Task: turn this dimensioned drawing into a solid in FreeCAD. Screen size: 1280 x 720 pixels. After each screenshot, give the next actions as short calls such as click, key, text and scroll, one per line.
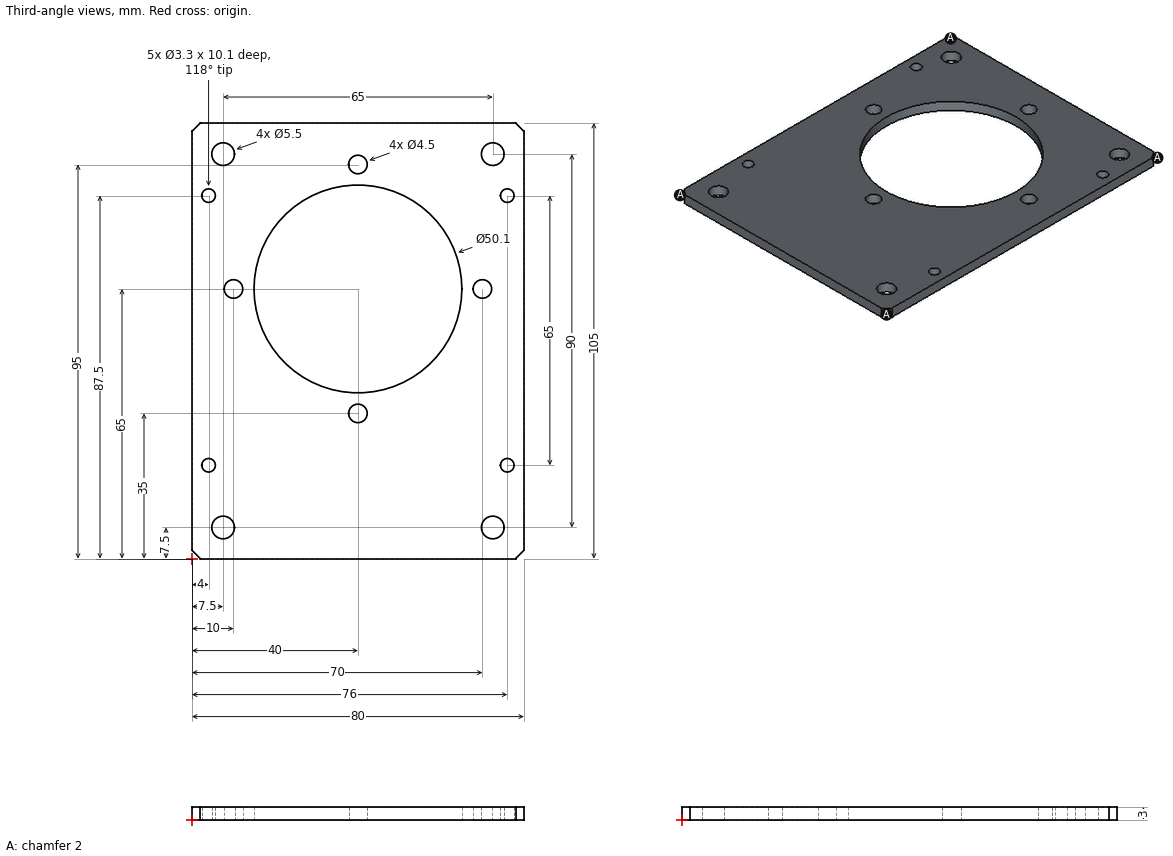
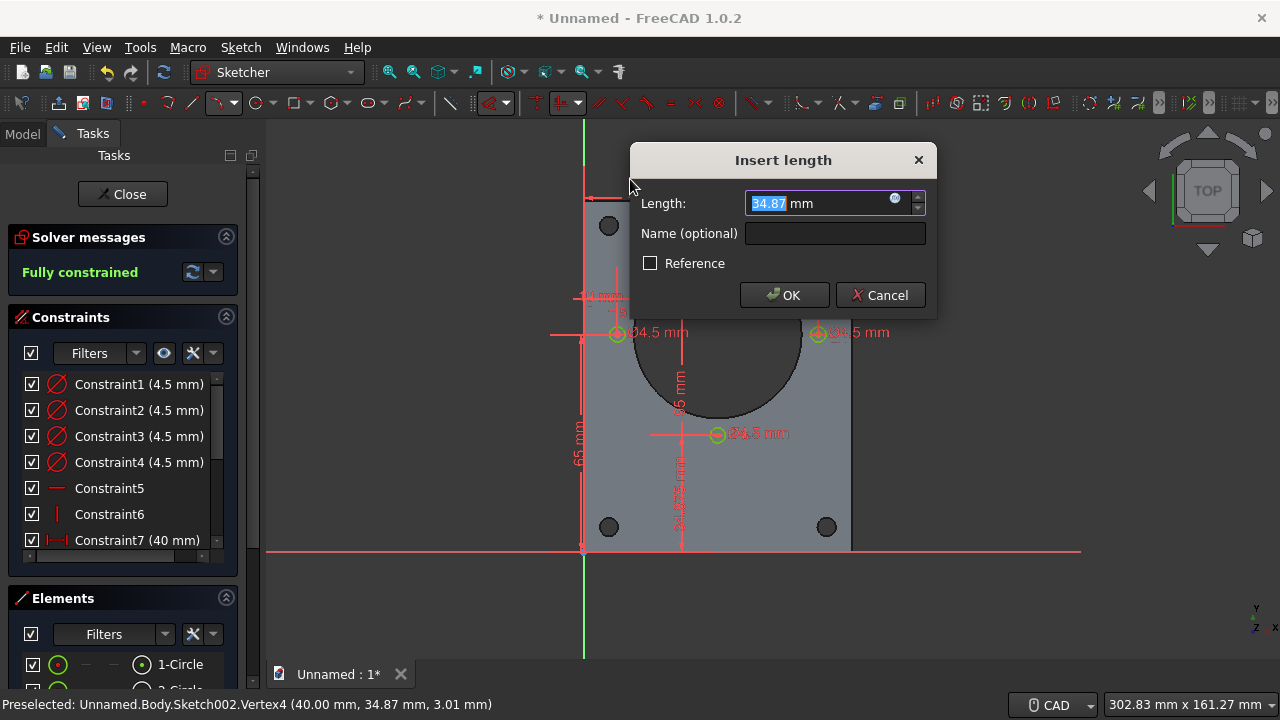
text(35)
key(Return)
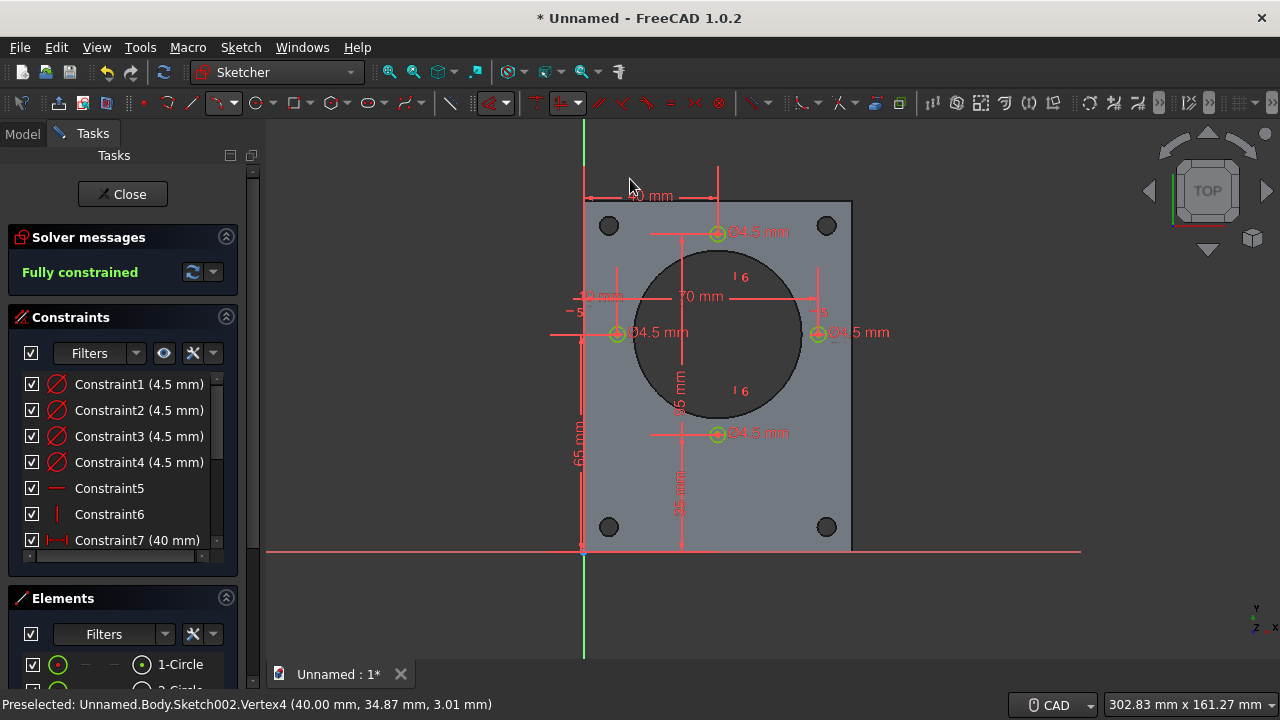
click(123, 194)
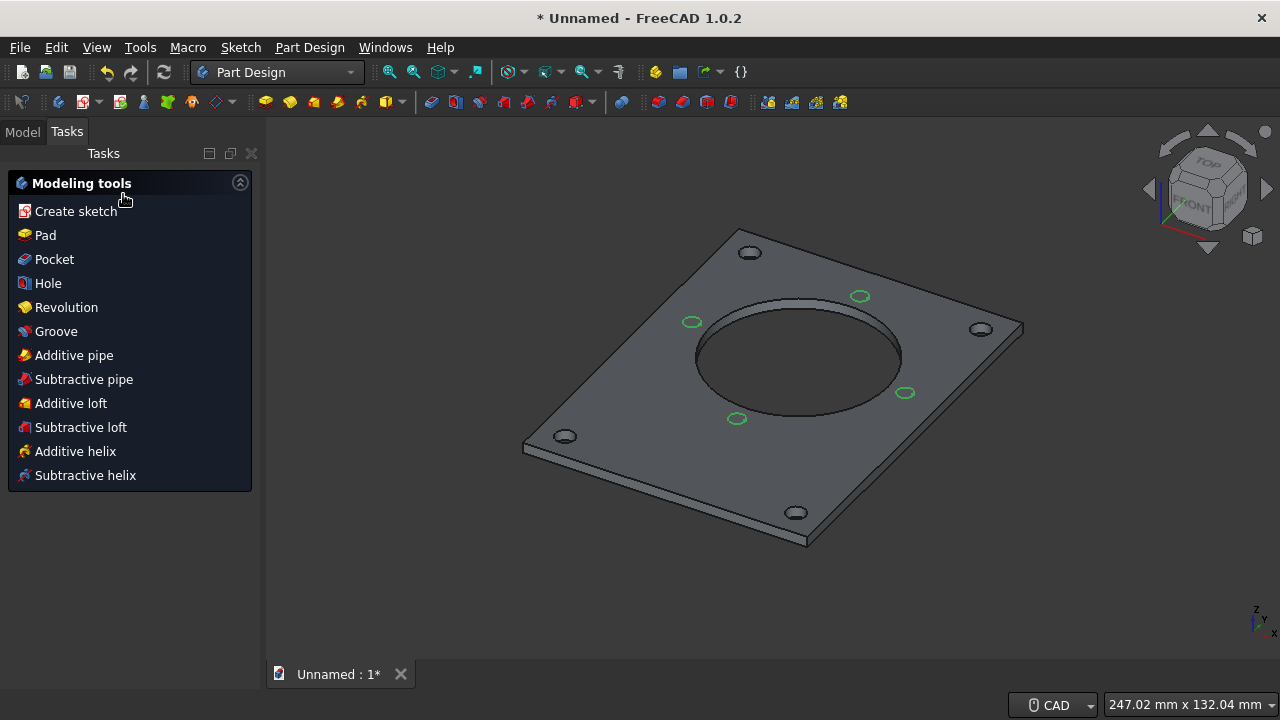
click(432, 102)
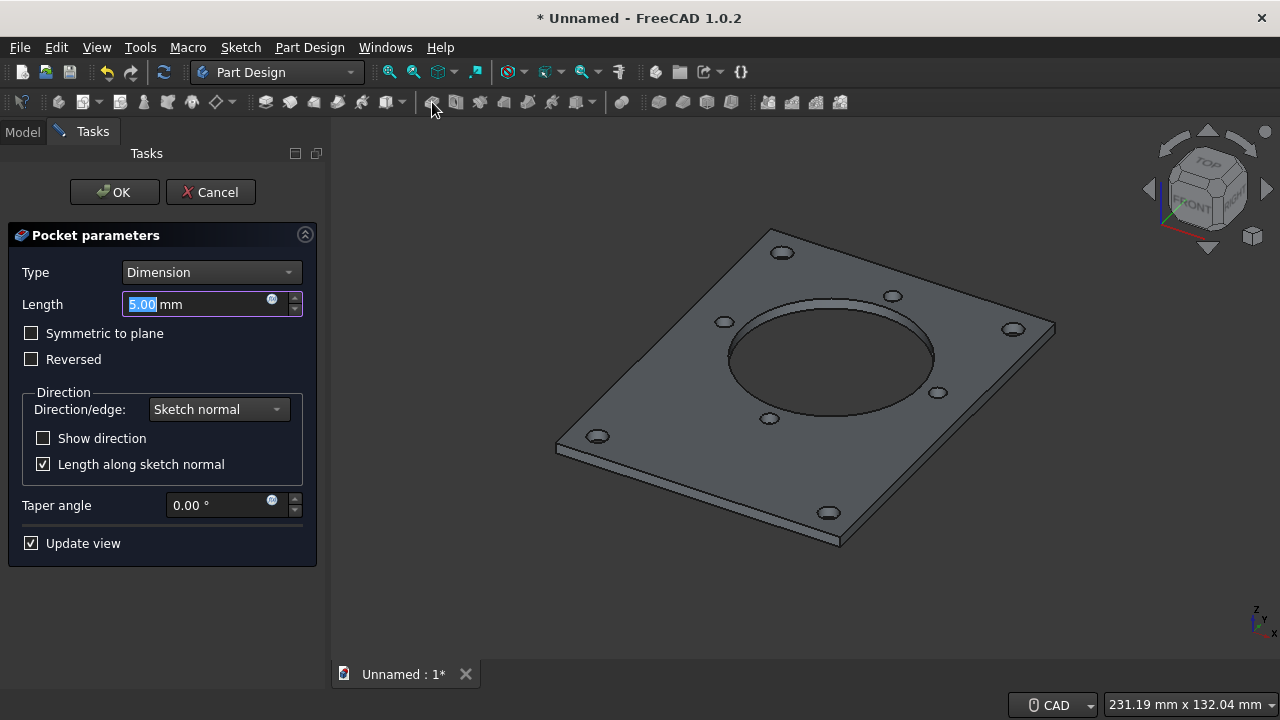
click(212, 272)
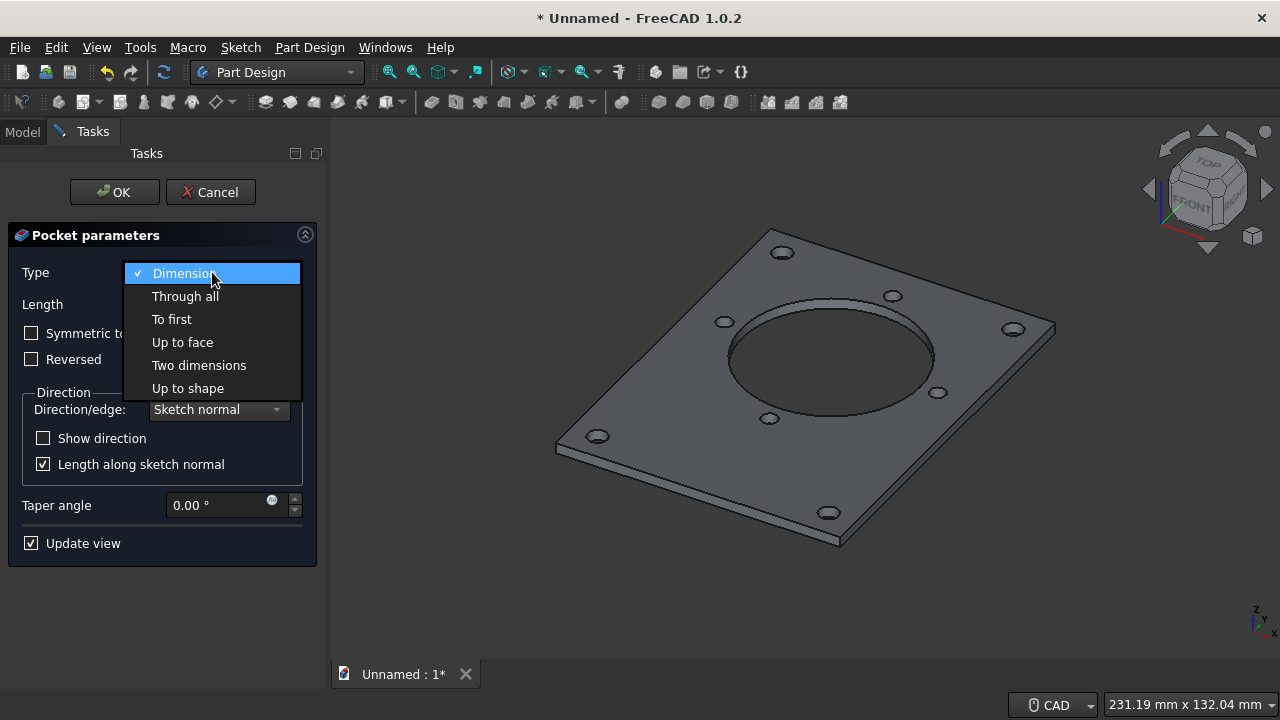
click(212, 296)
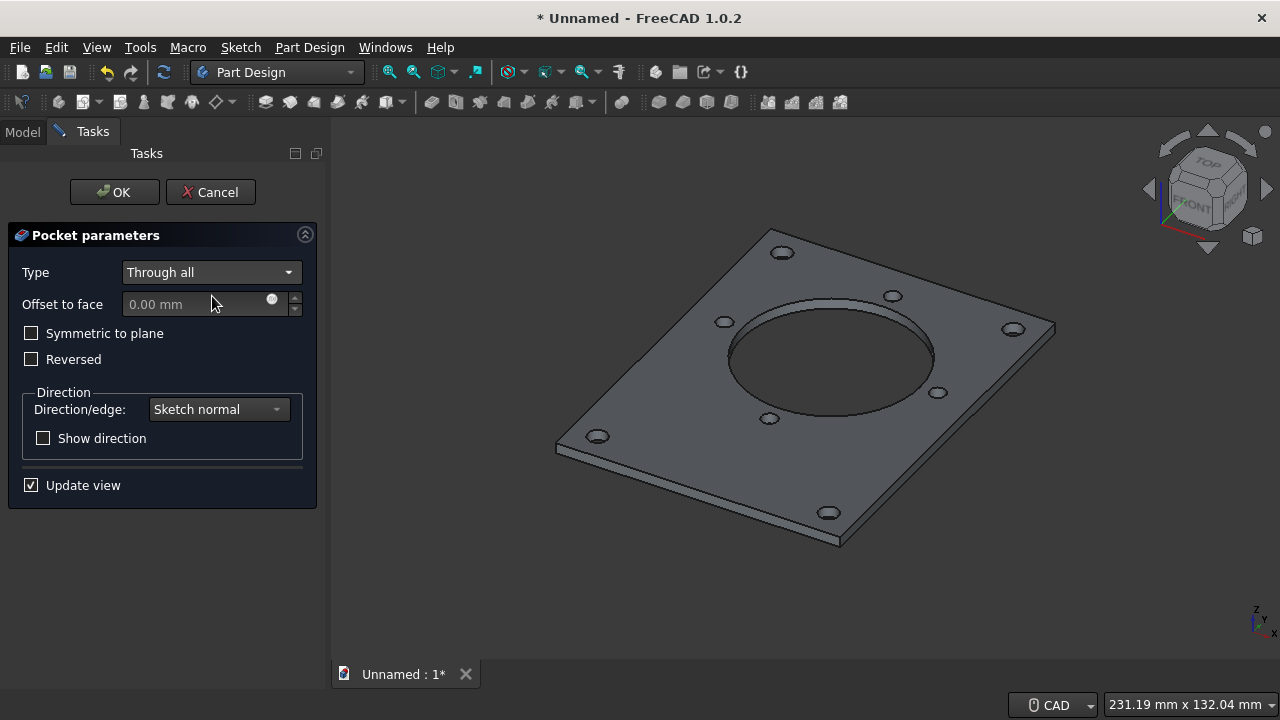
click(115, 192)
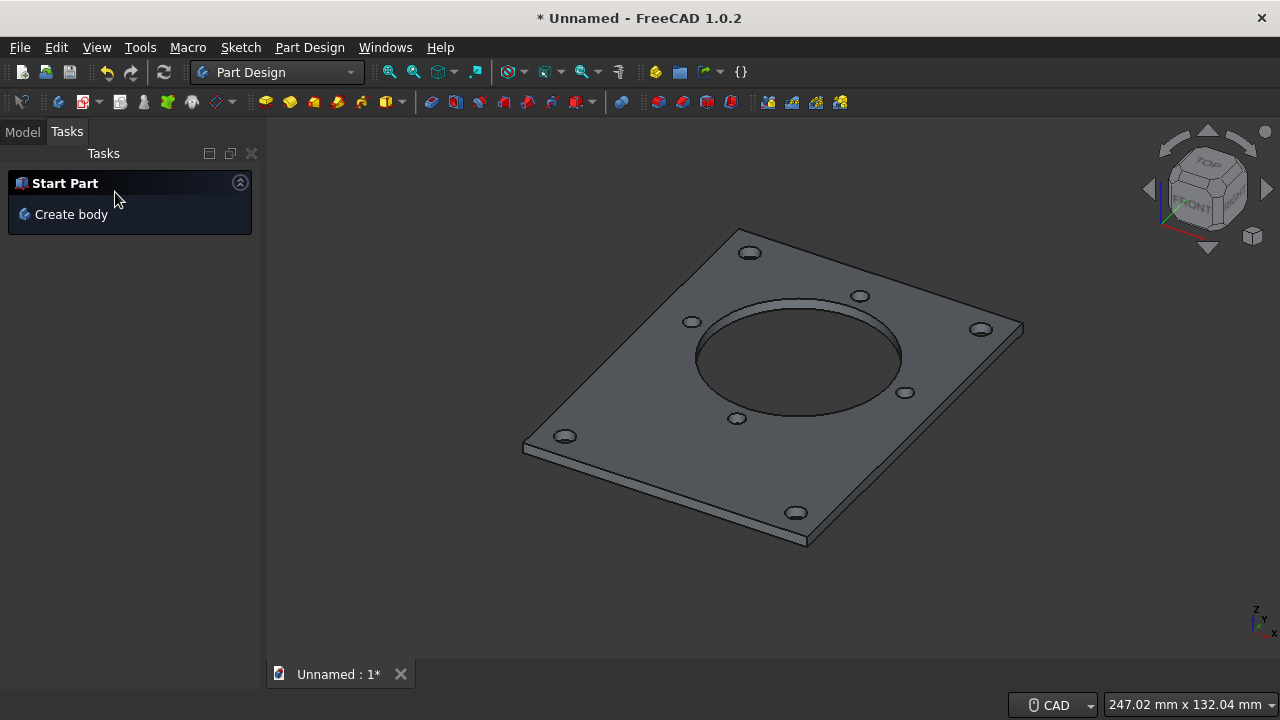
click(807, 543)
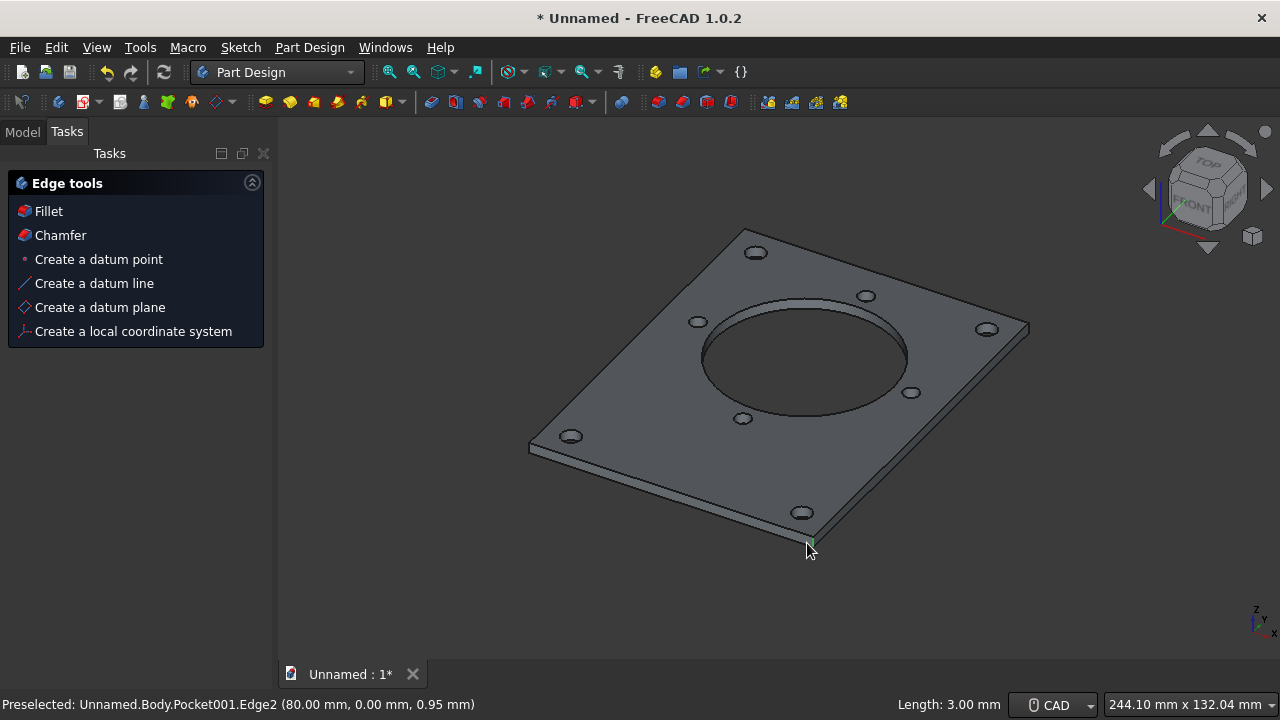
scroll(745, 233, up, 6)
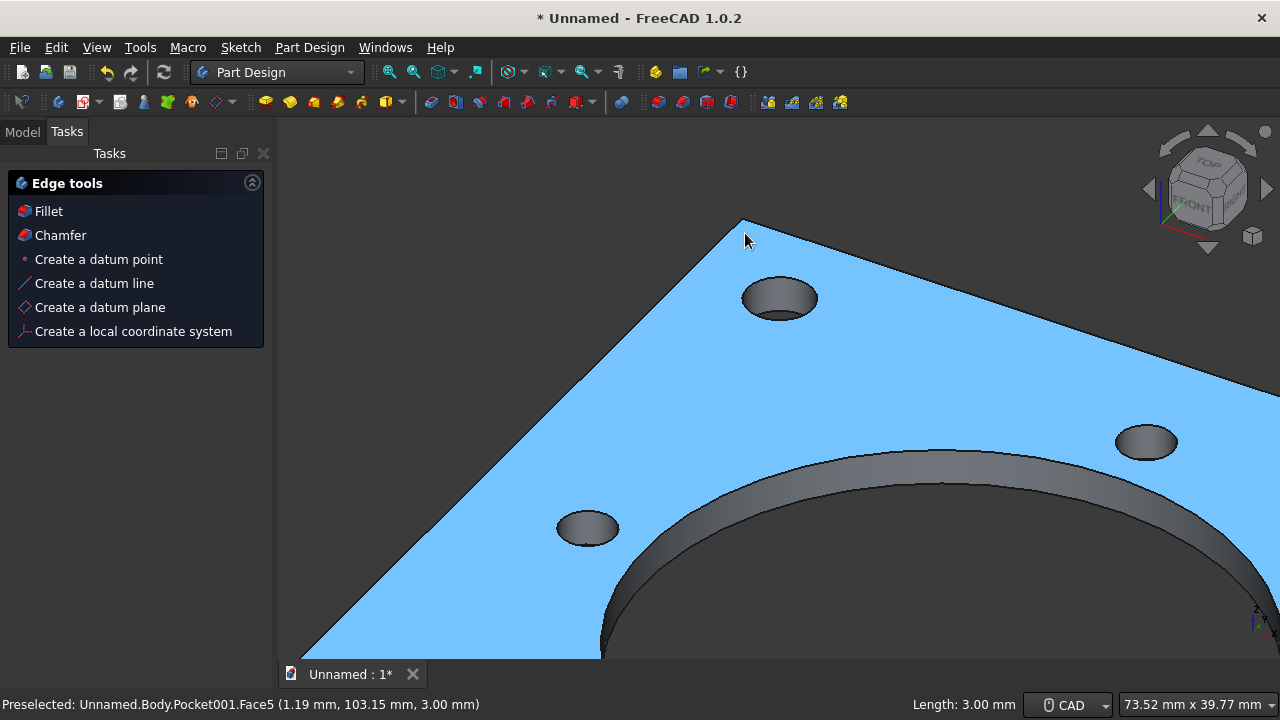
click(390, 72)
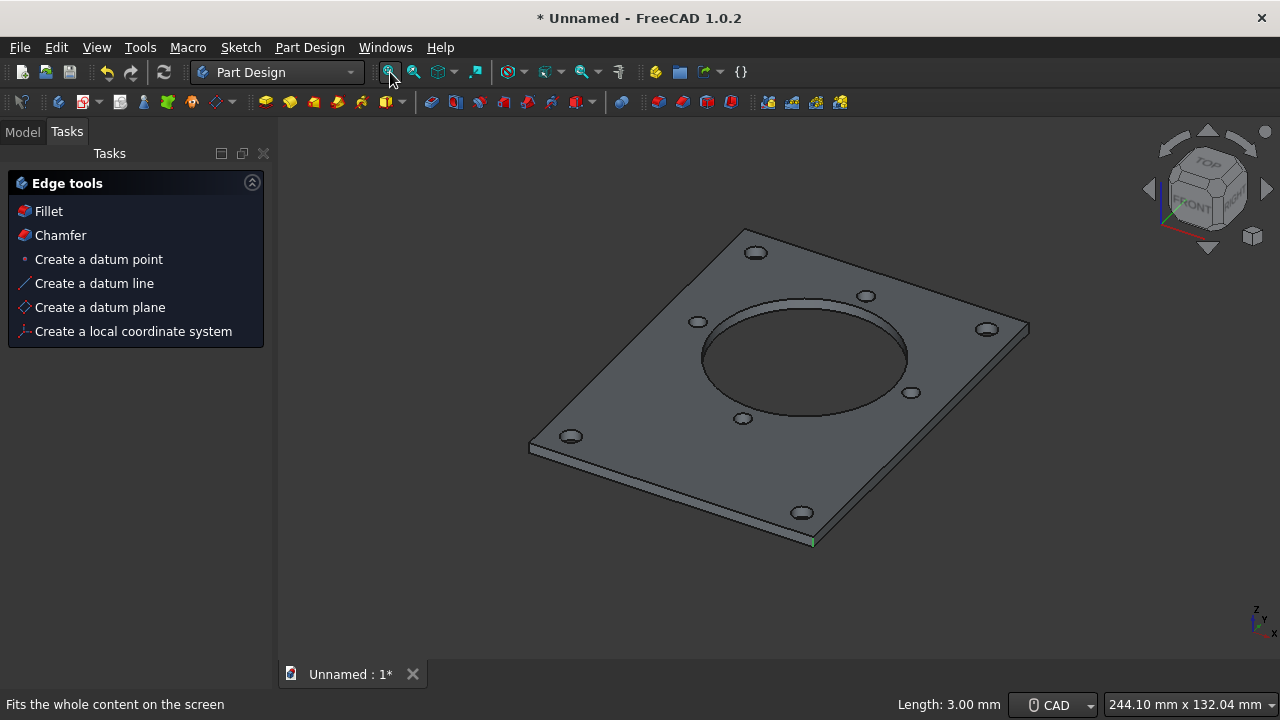
key(0)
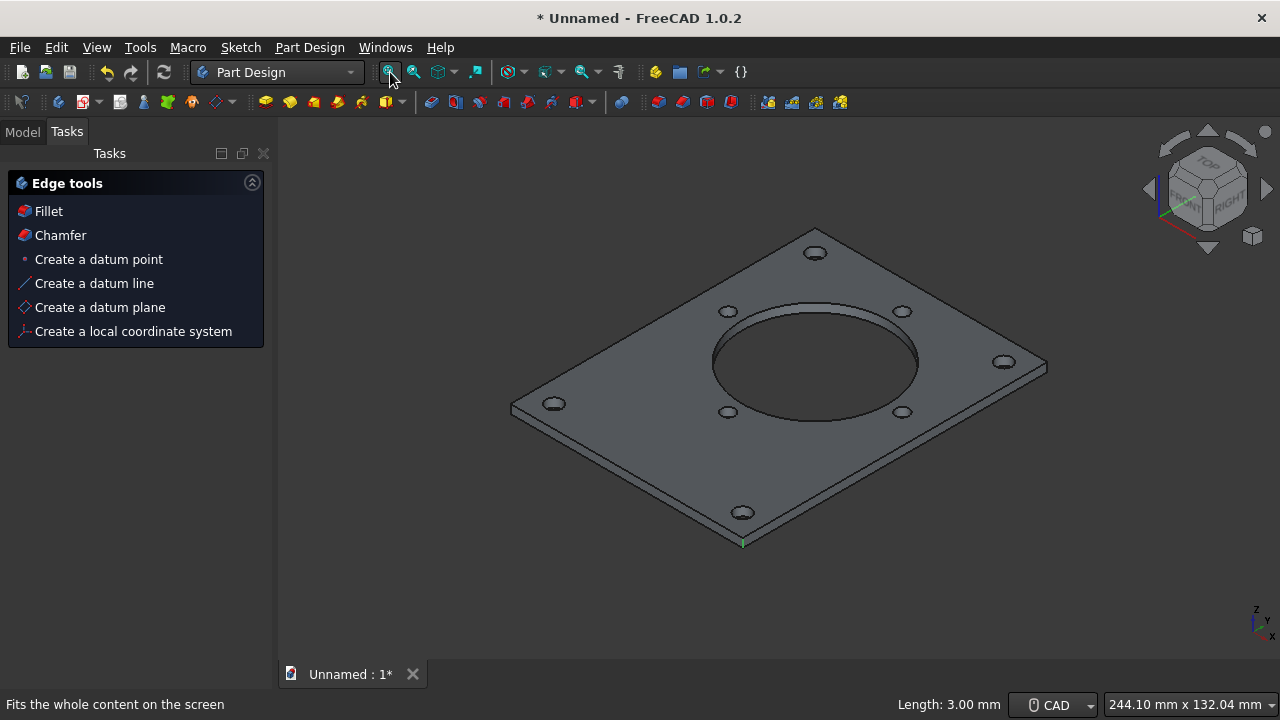
scroll(815, 232, up, 6)